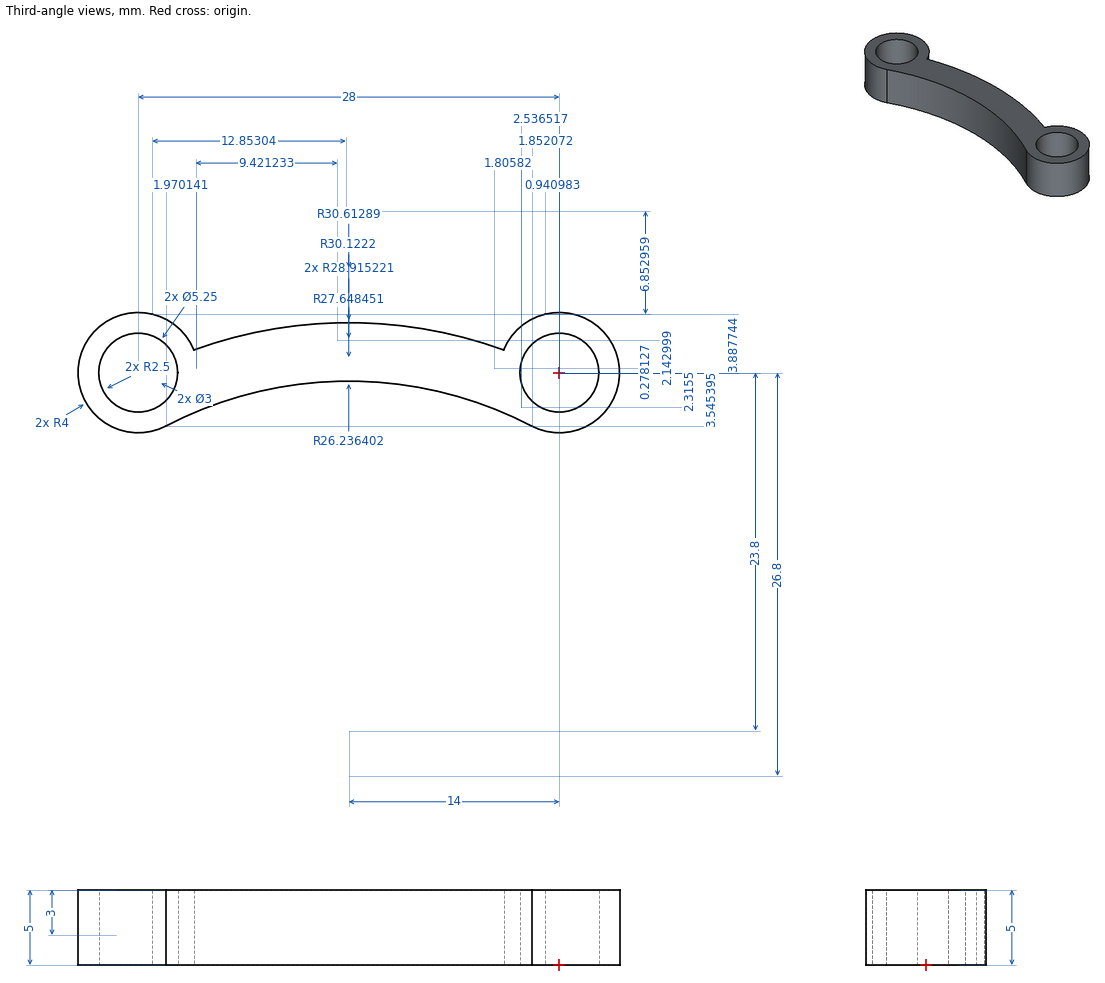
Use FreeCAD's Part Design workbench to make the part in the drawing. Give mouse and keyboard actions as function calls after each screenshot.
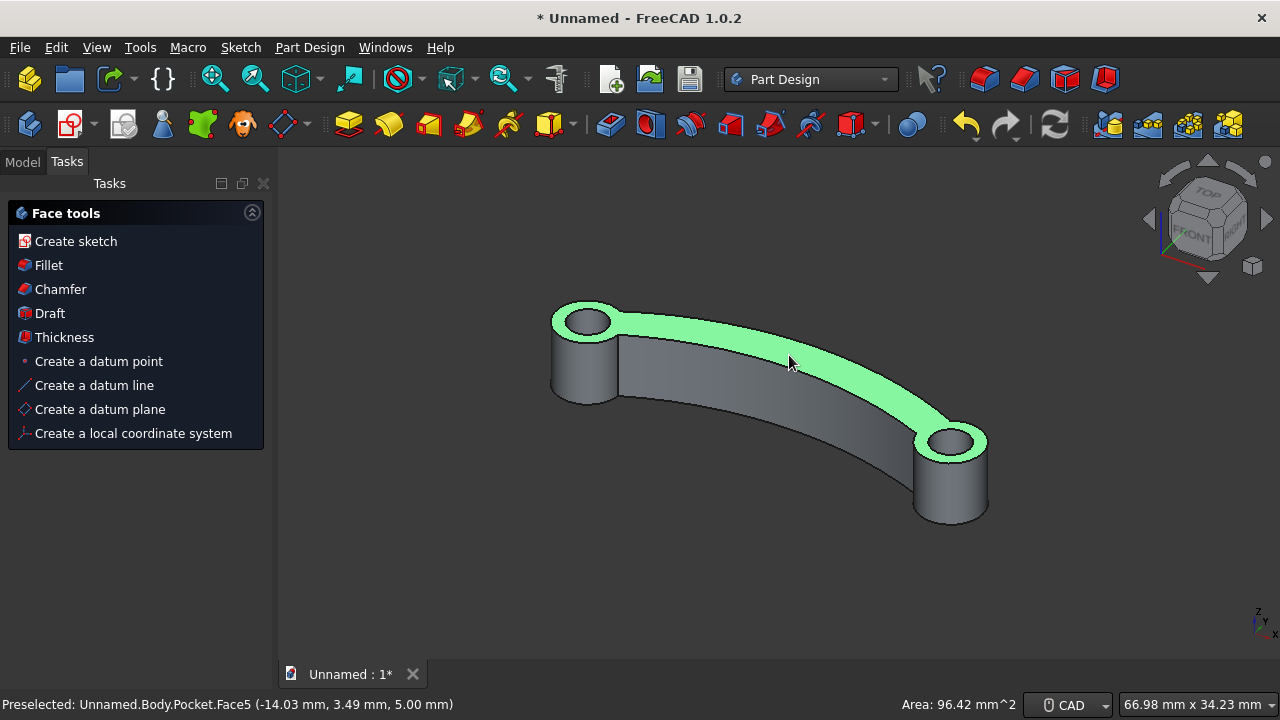
click(70, 124)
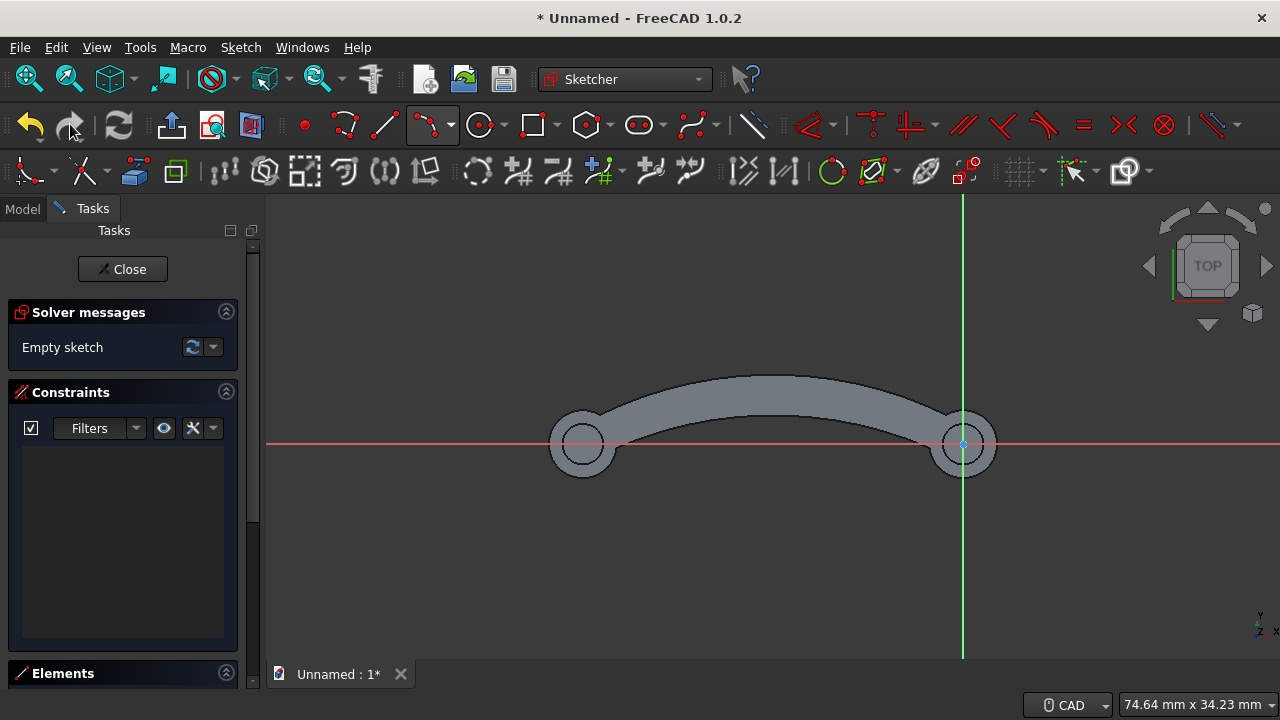
key(g)
key(3)
key(a)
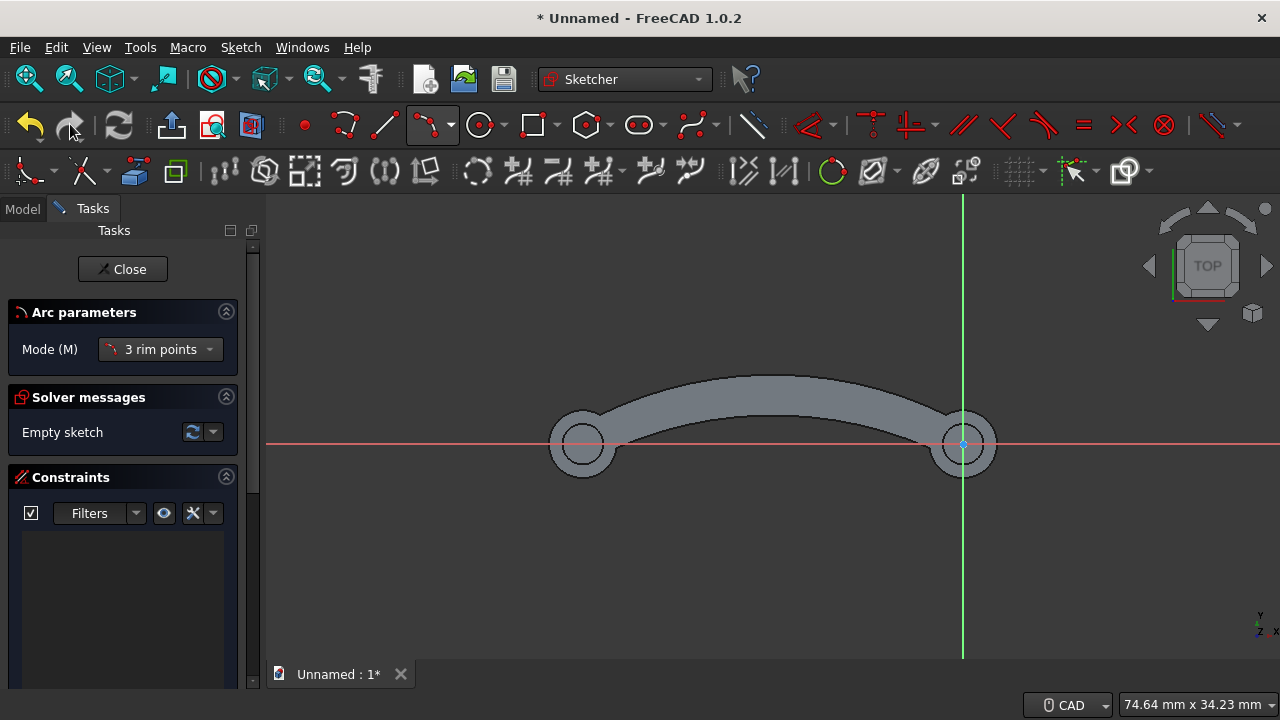
click(911, 459)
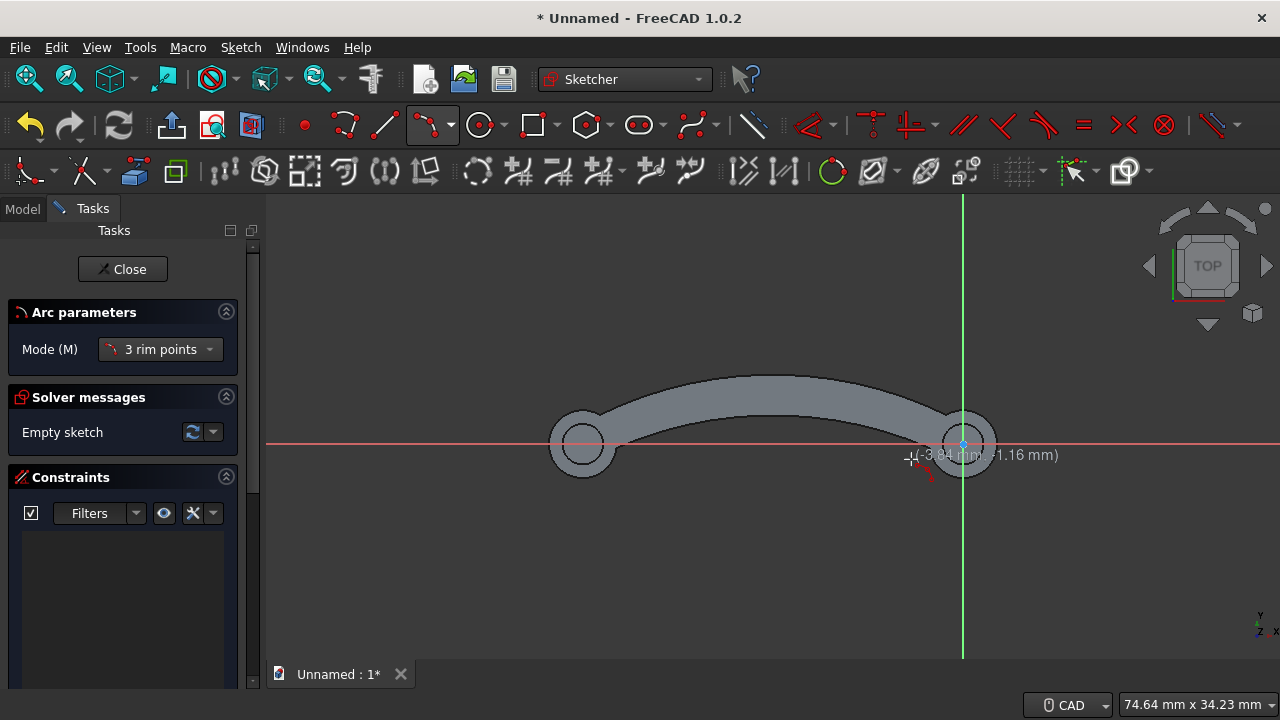
scroll(950, 391, up, 2)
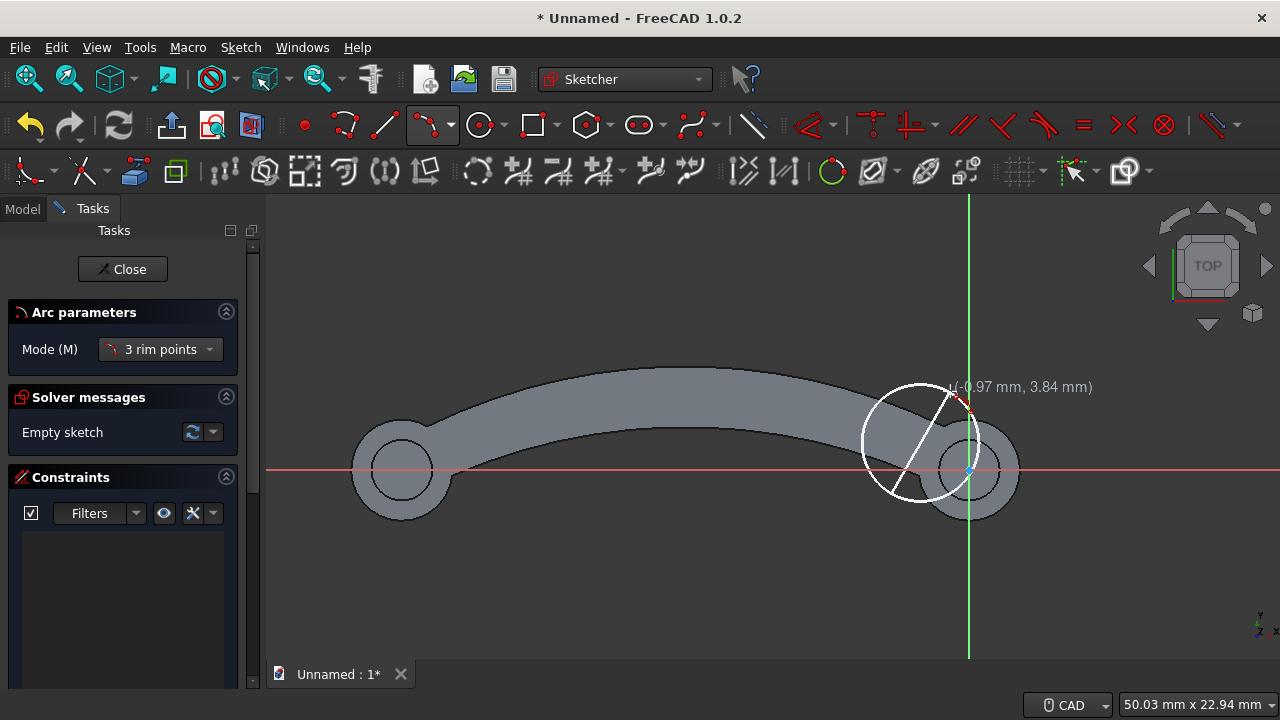
click(950, 391)
click(1039, 511)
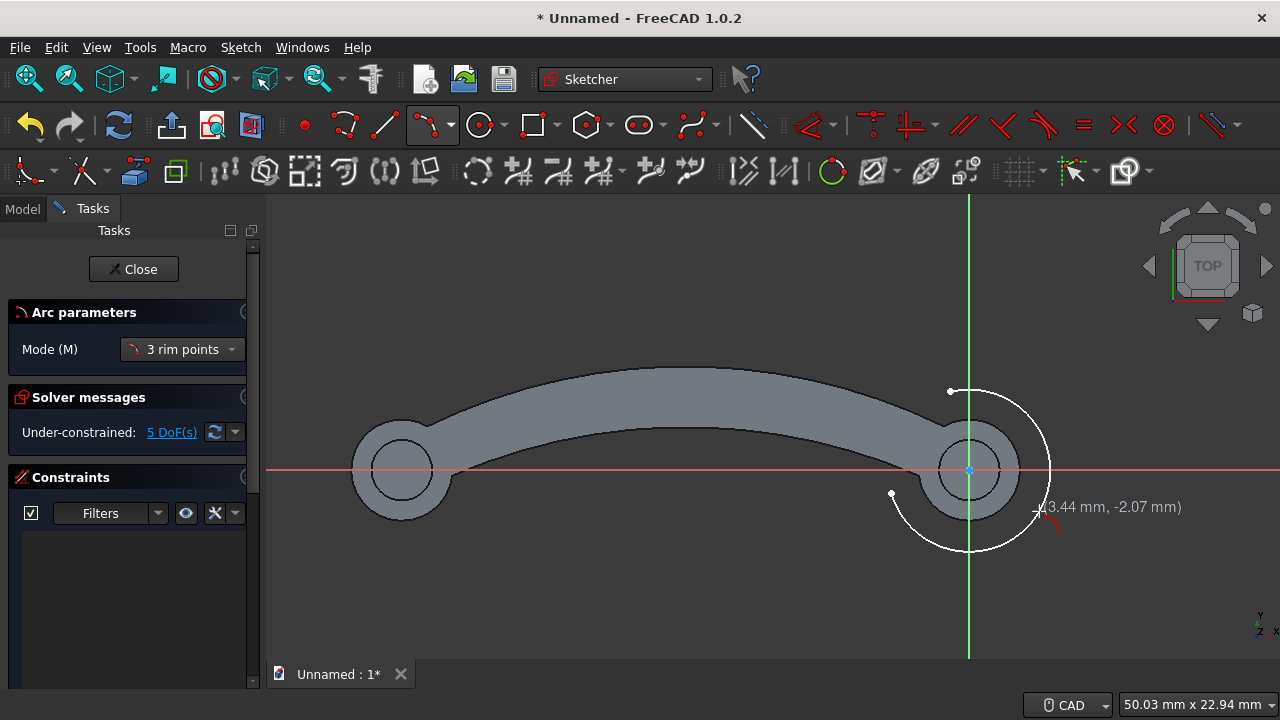
click(950, 392)
click(421, 391)
click(686, 332)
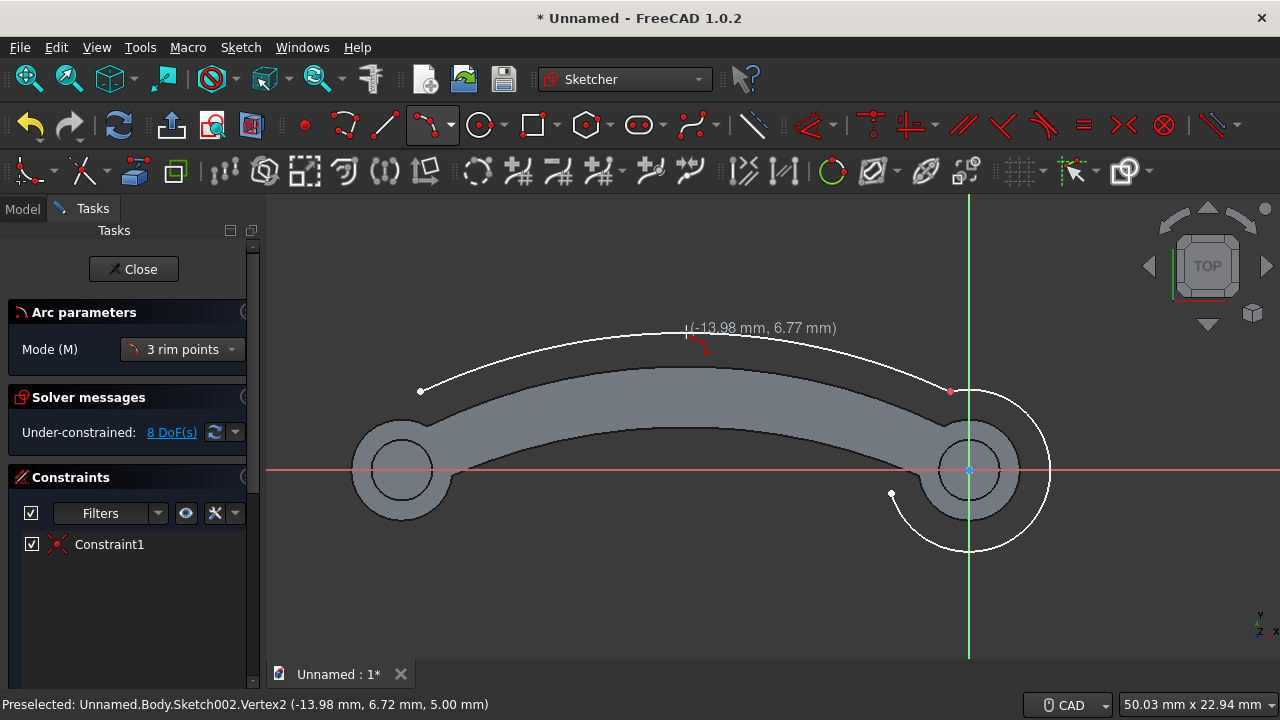
click(421, 392)
click(480, 492)
click(332, 511)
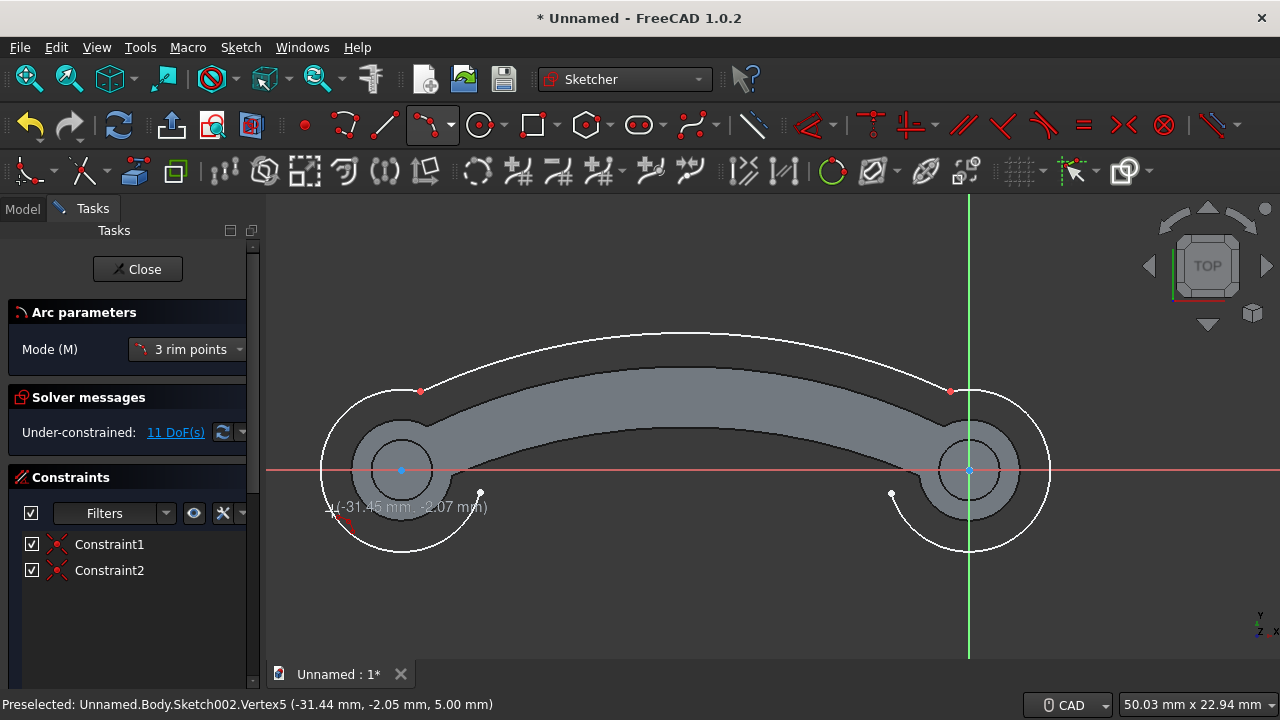
click(480, 493)
click(891, 494)
click(686, 453)
key(Escape)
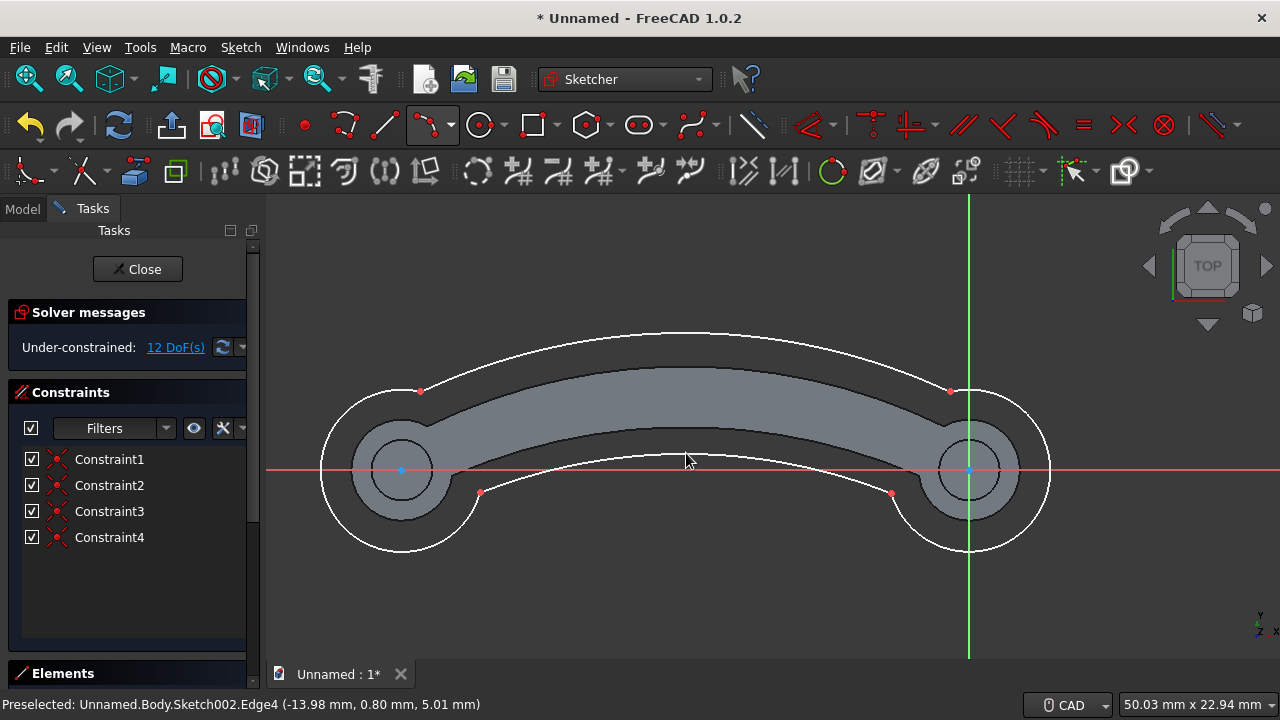
drag(959, 460, 979, 481)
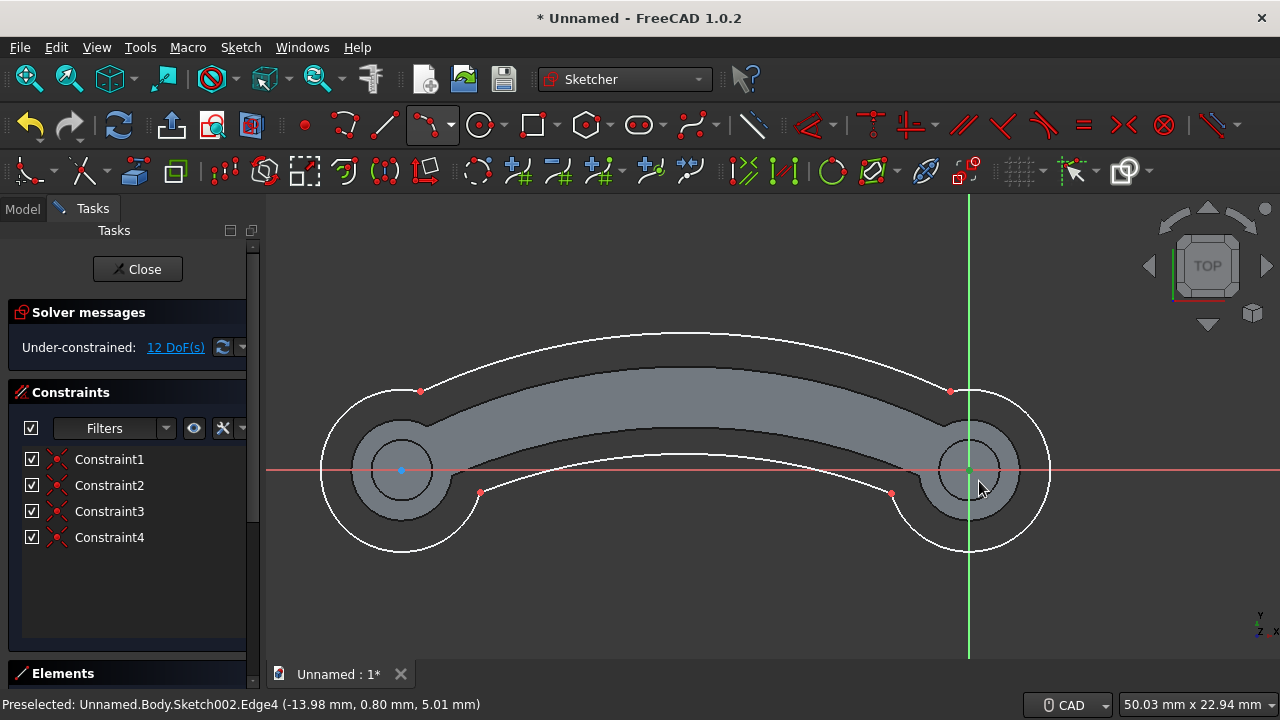
click(872, 126)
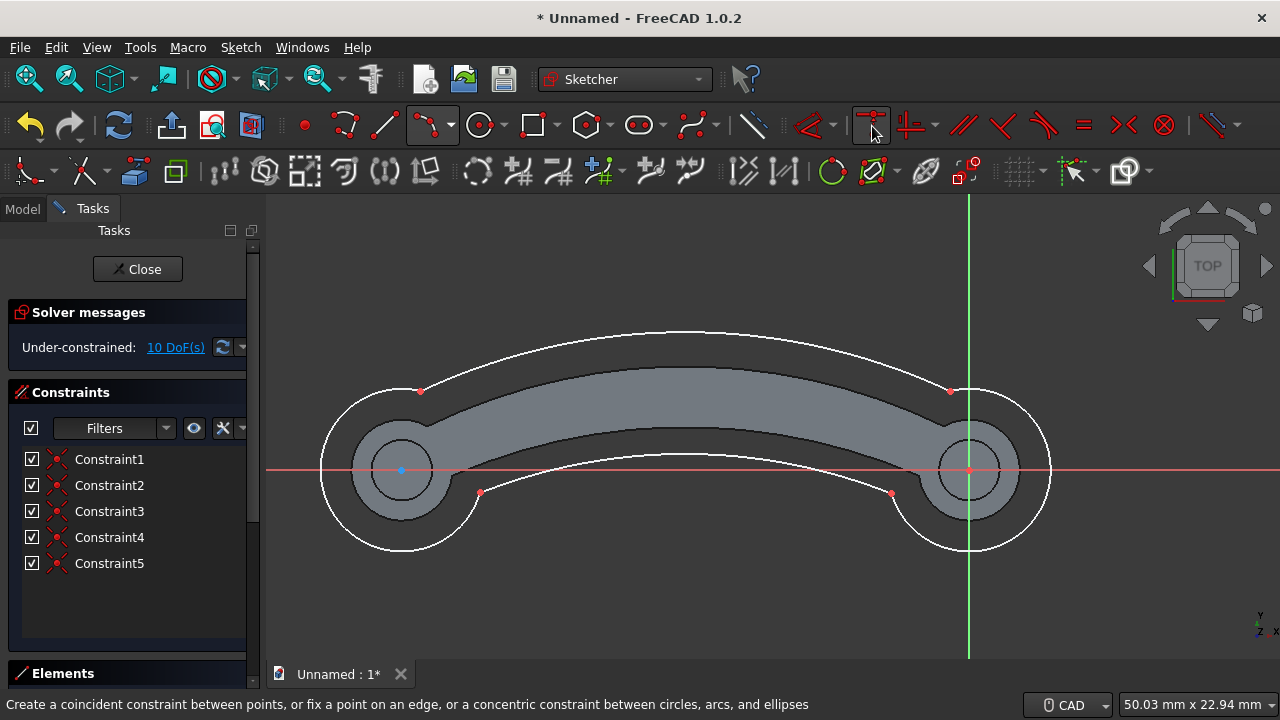
scroll(979, 551, up, 2)